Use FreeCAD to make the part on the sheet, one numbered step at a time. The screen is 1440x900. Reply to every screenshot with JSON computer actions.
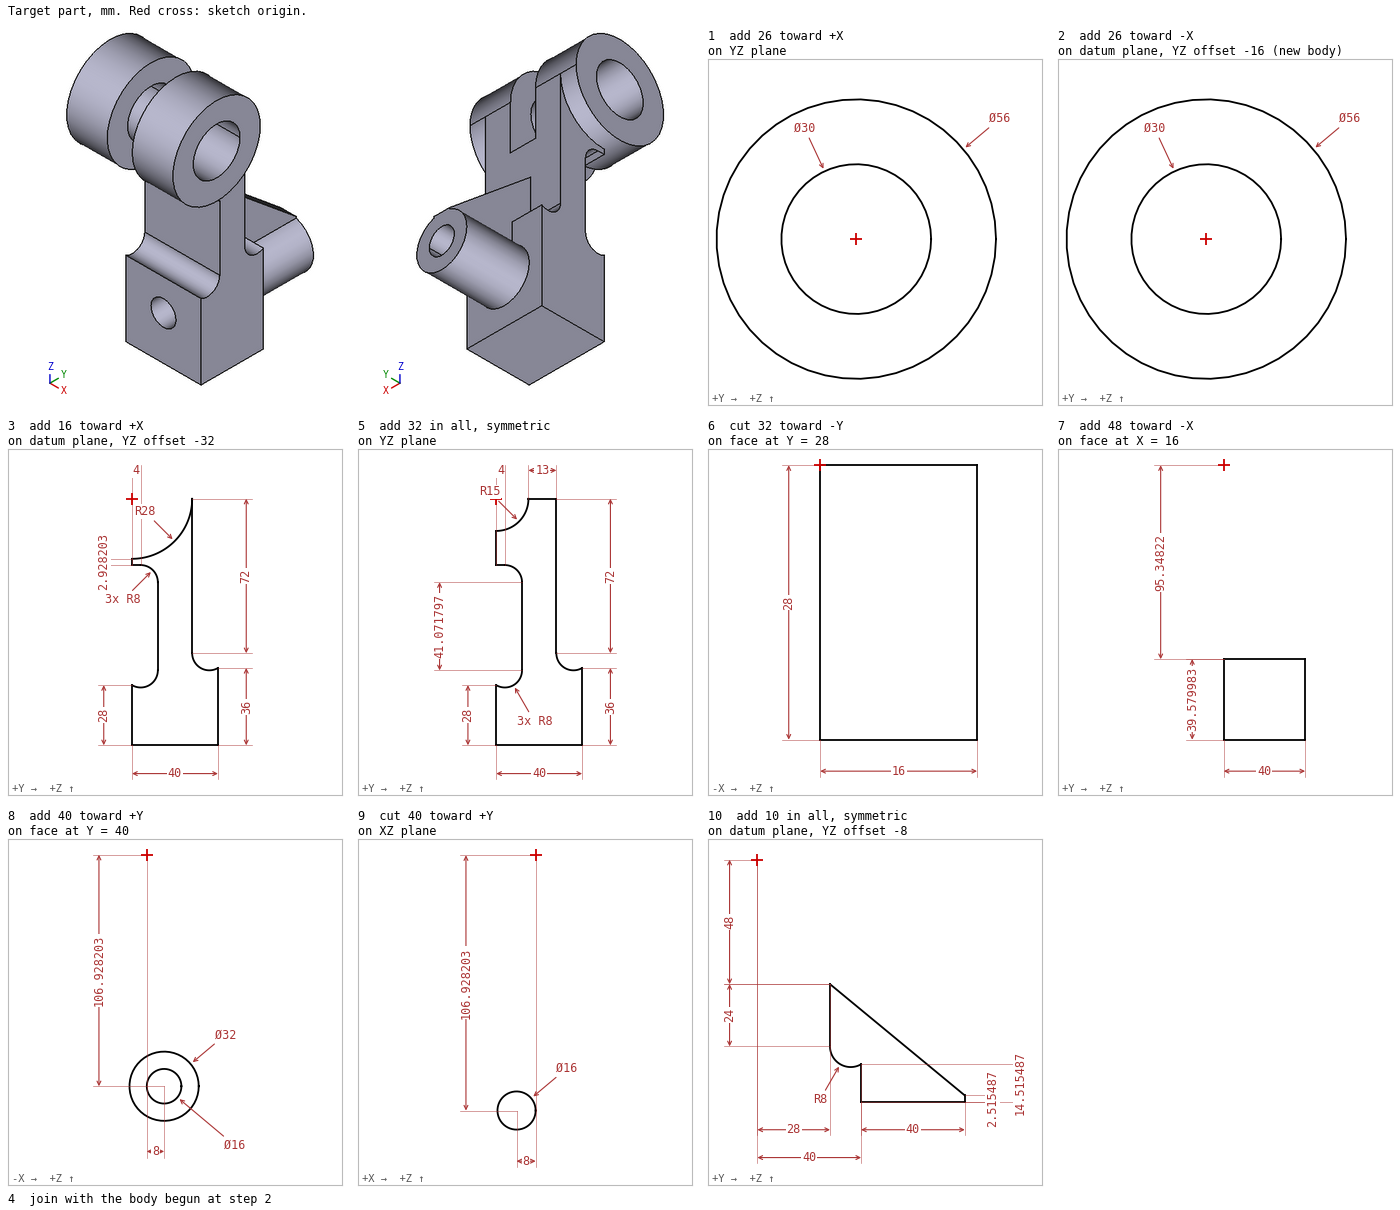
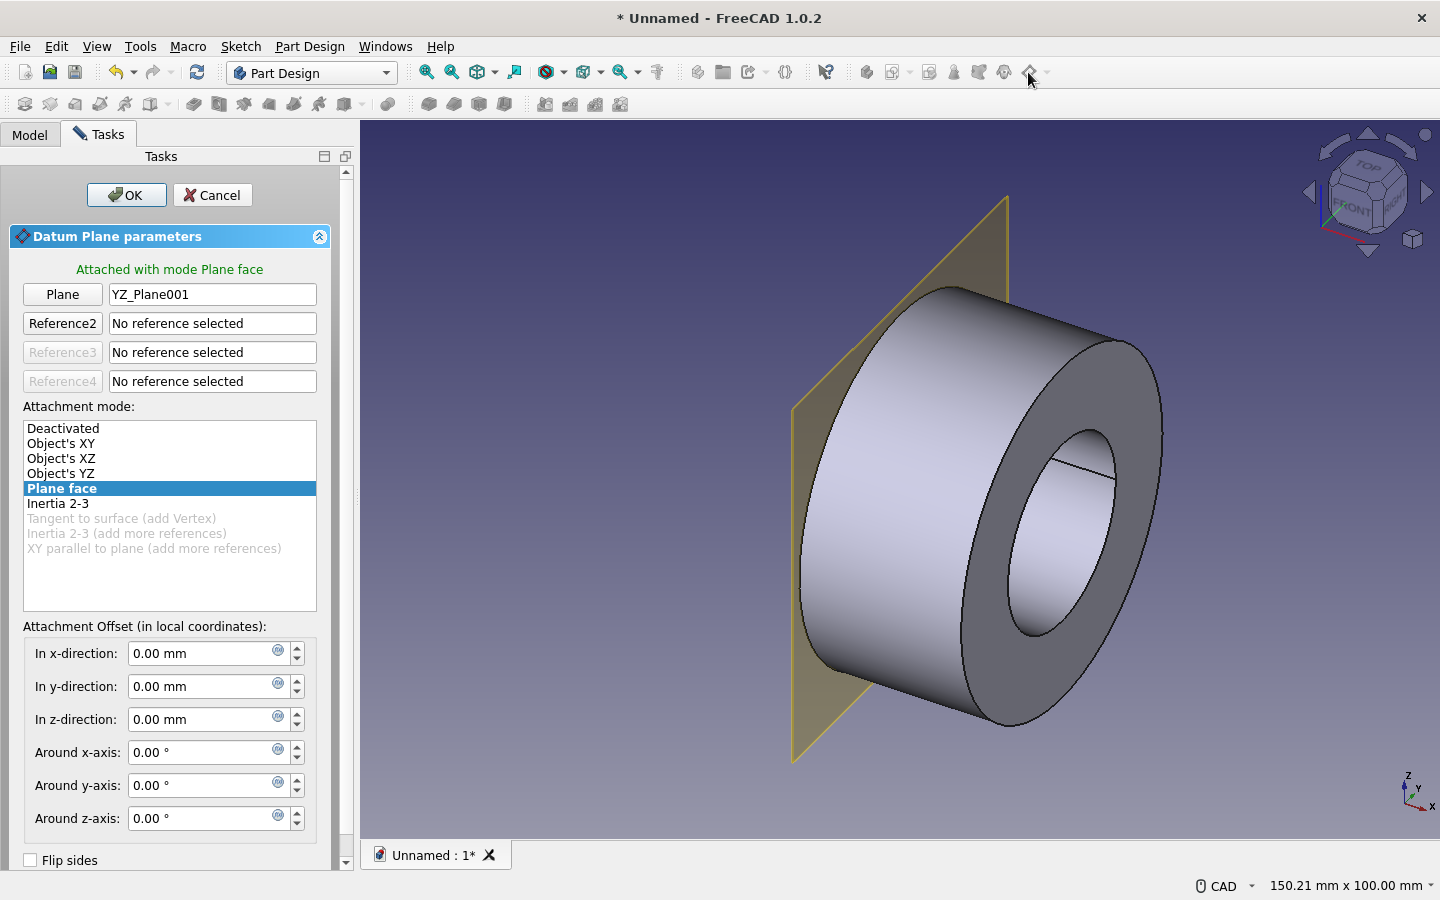
{"action": "triple_click", "coordinate": [210, 720]}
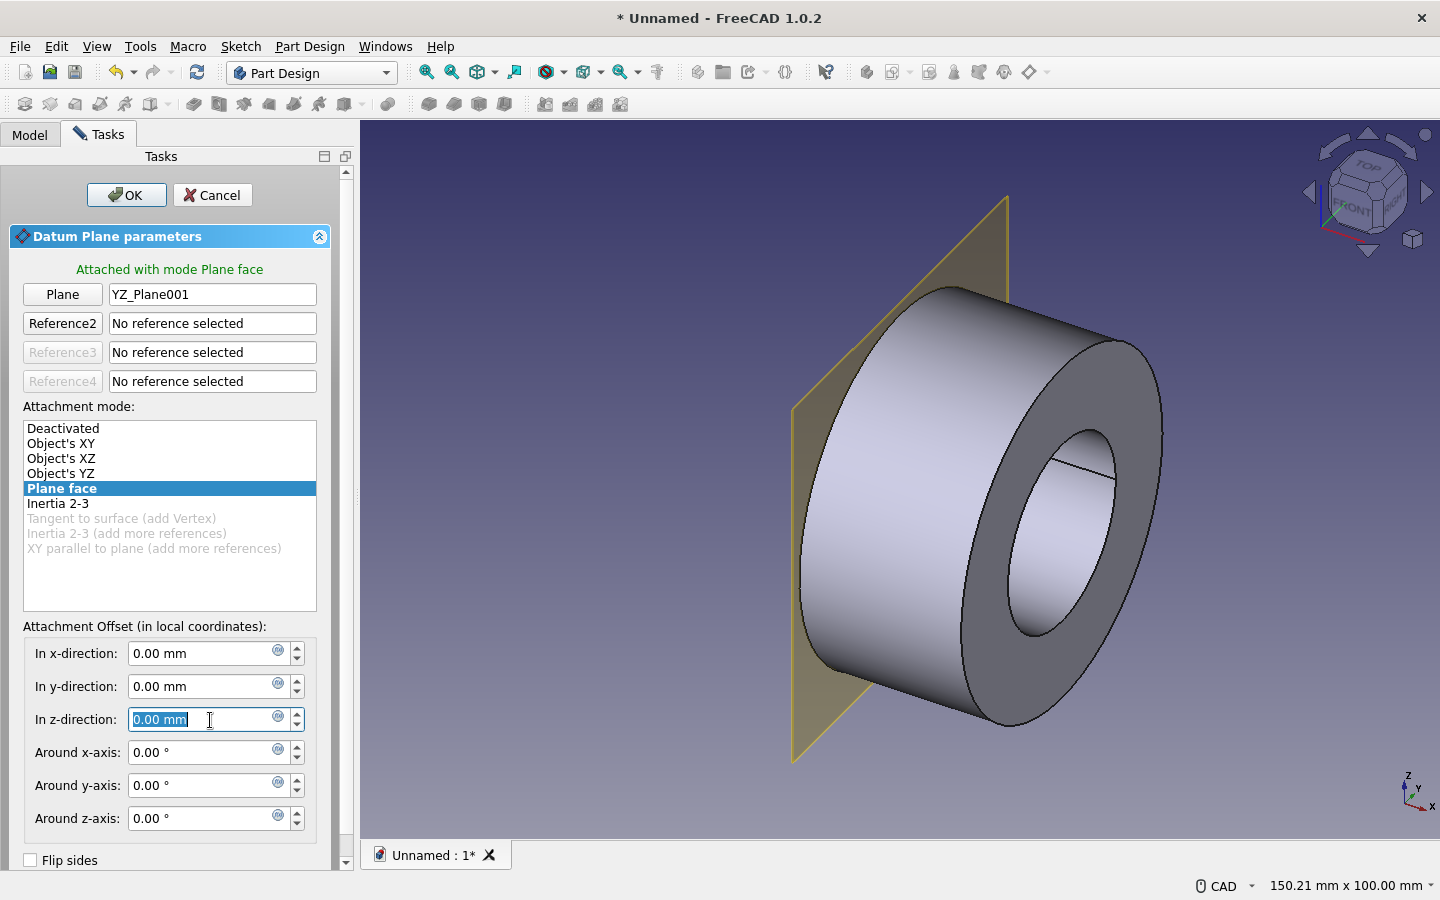
{"action": "type", "text": "-16"}
{"action": "key", "text": "Tab"}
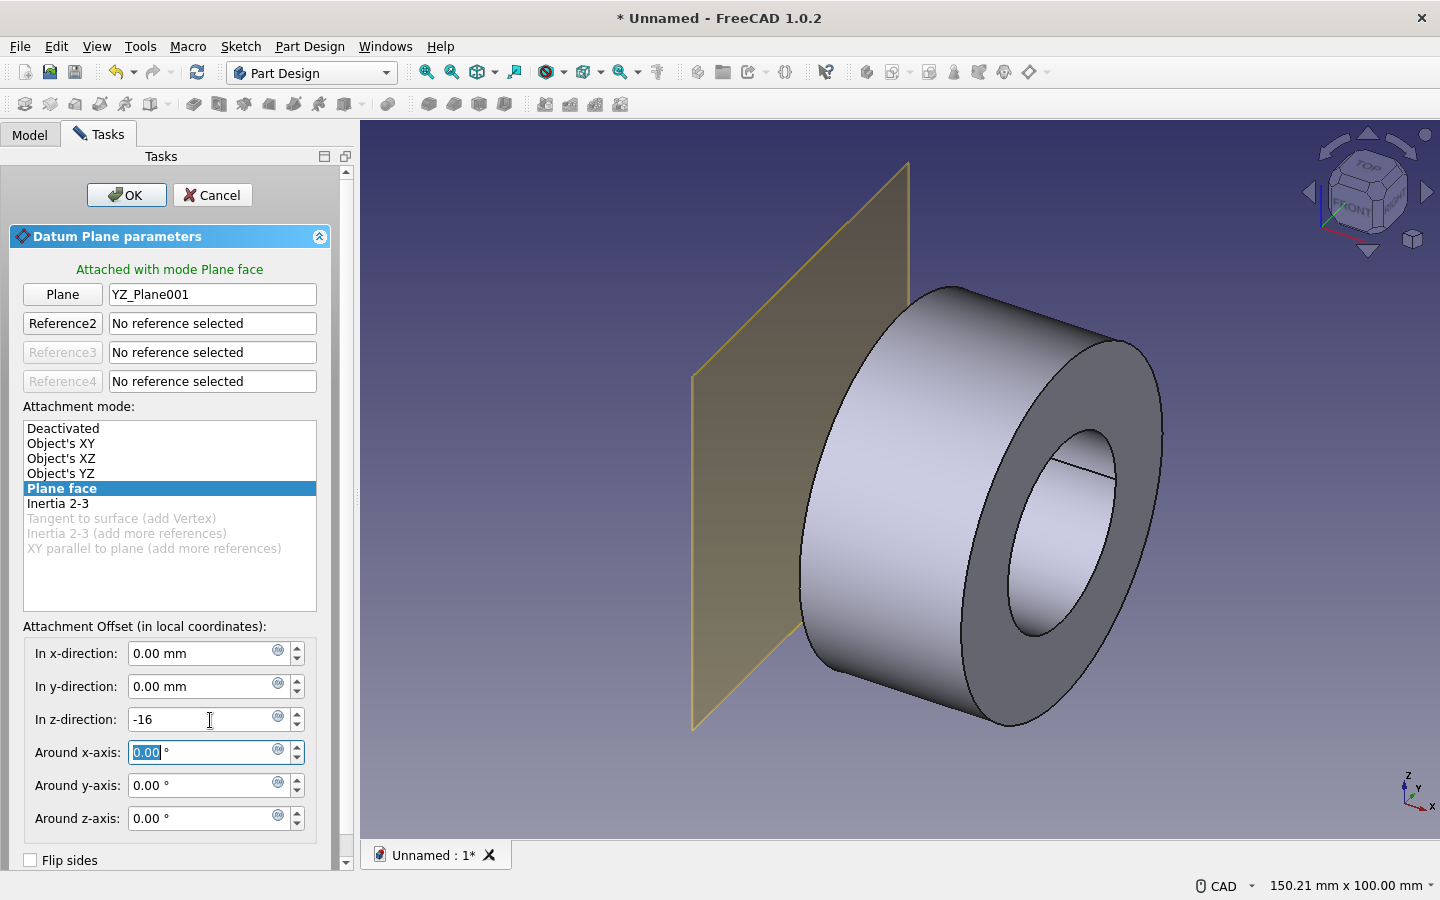
{"action": "left_click", "coordinate": [127, 195]}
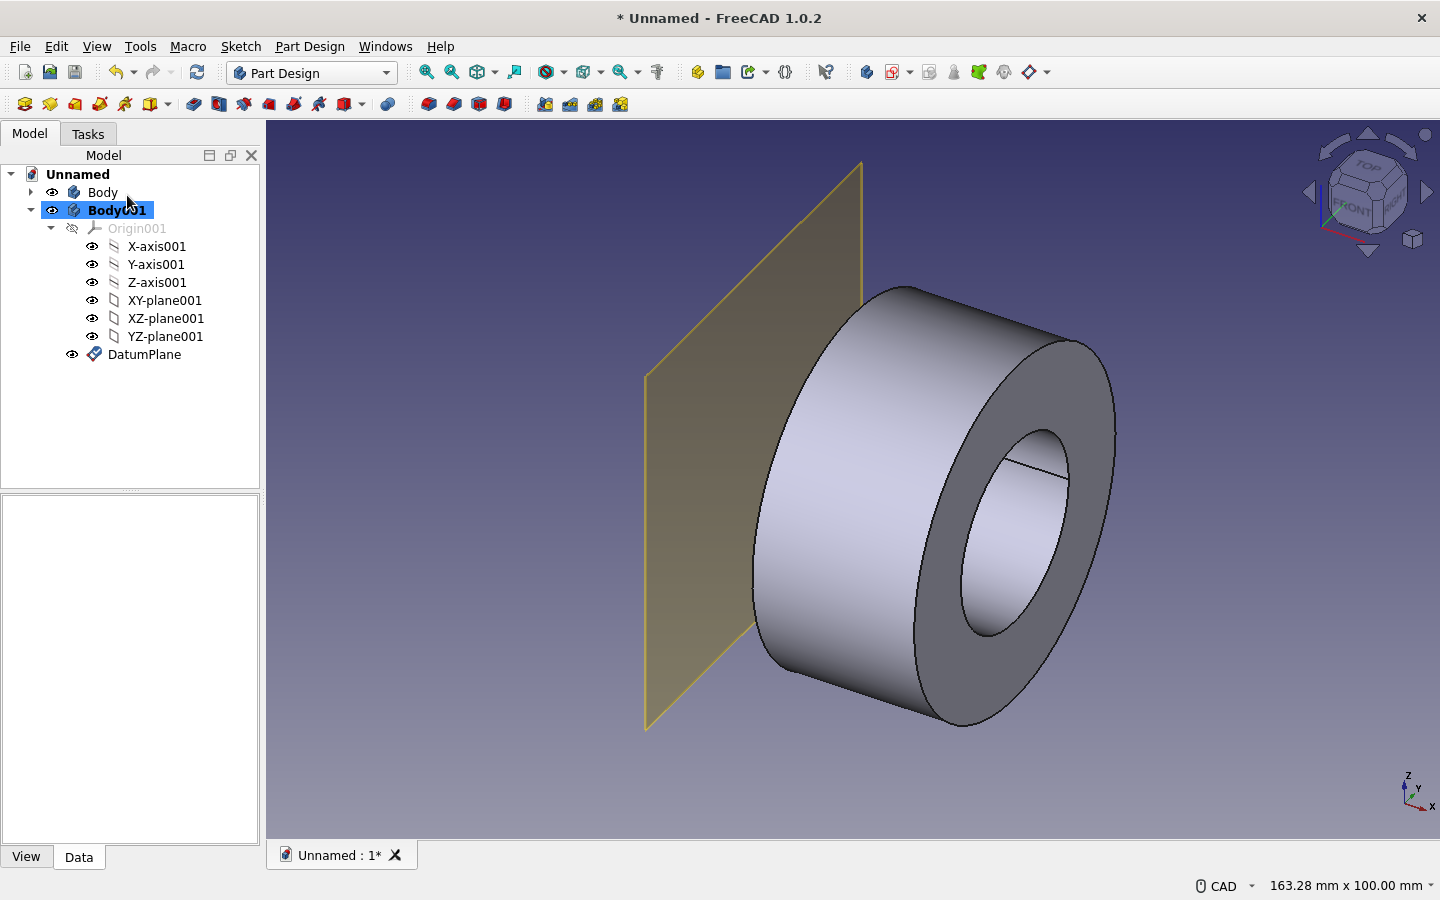
{"action": "left_click", "coordinate": [117, 354]}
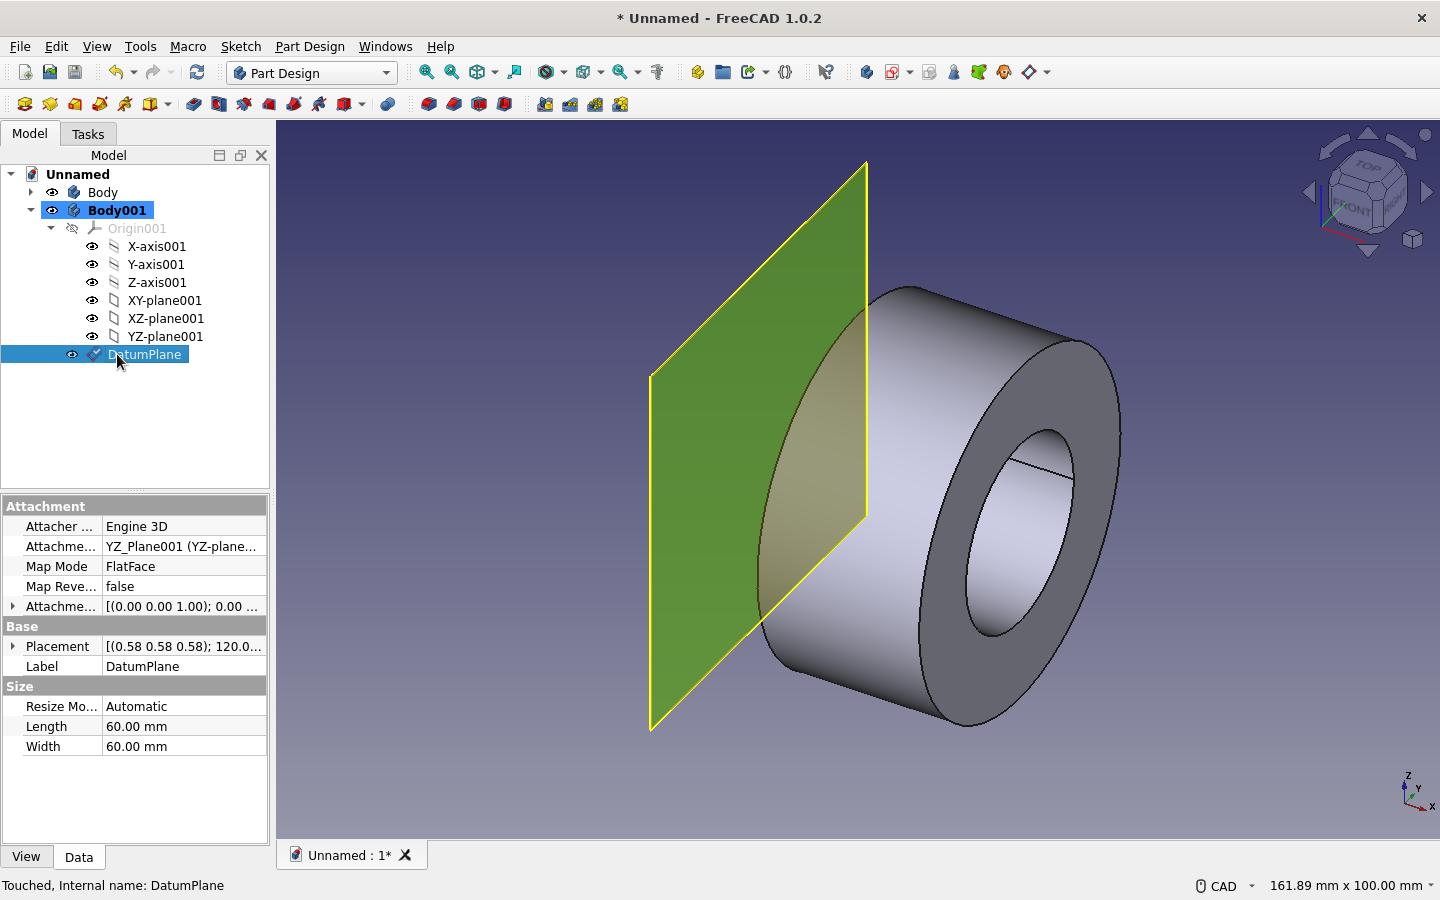
{"action": "left_click", "coordinate": [892, 72]}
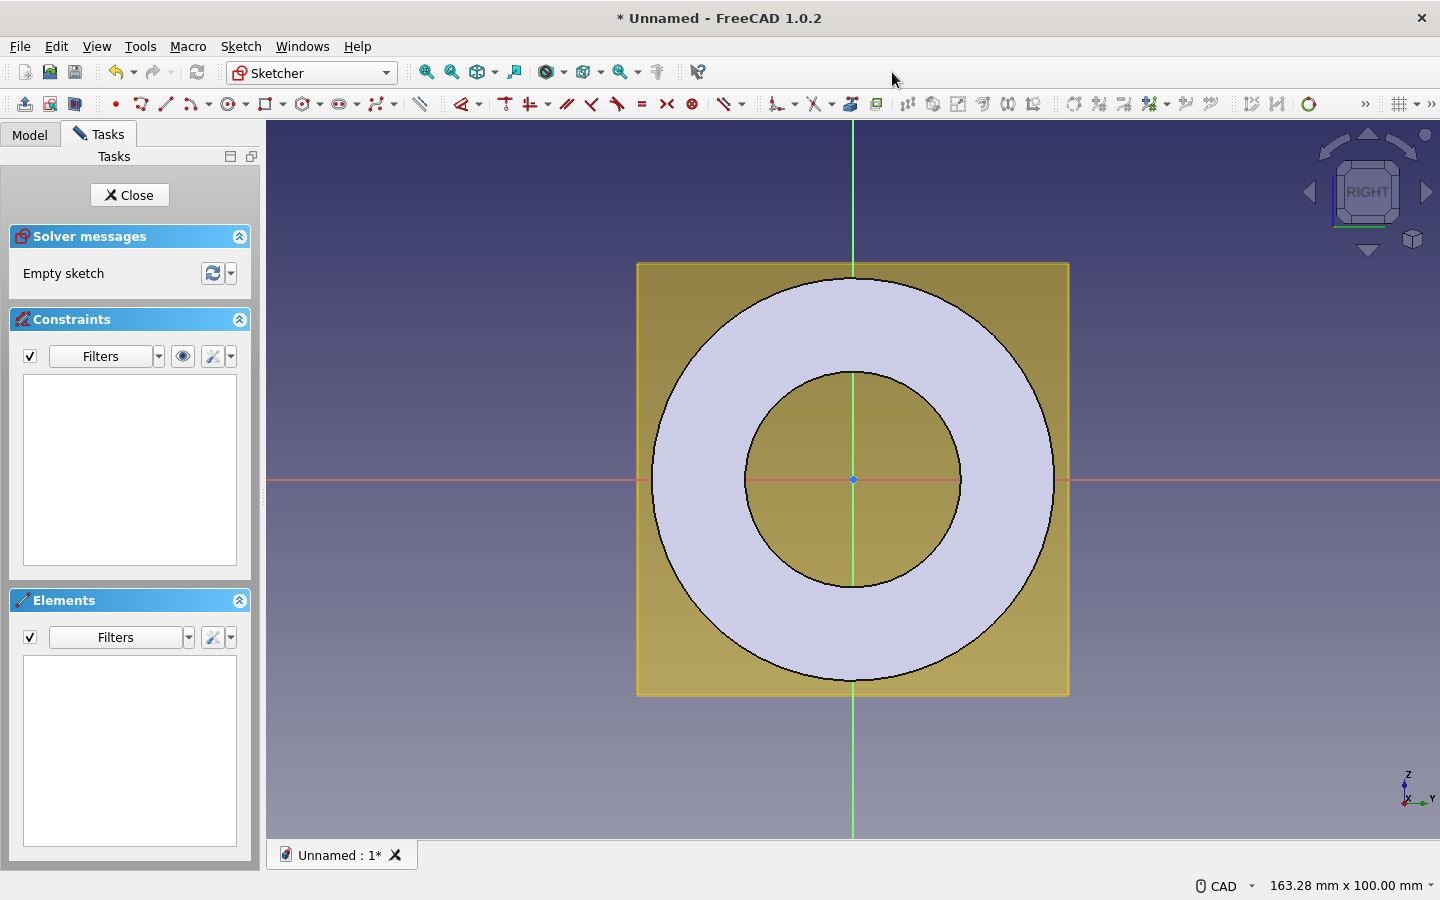
{"action": "key", "text": "g c"}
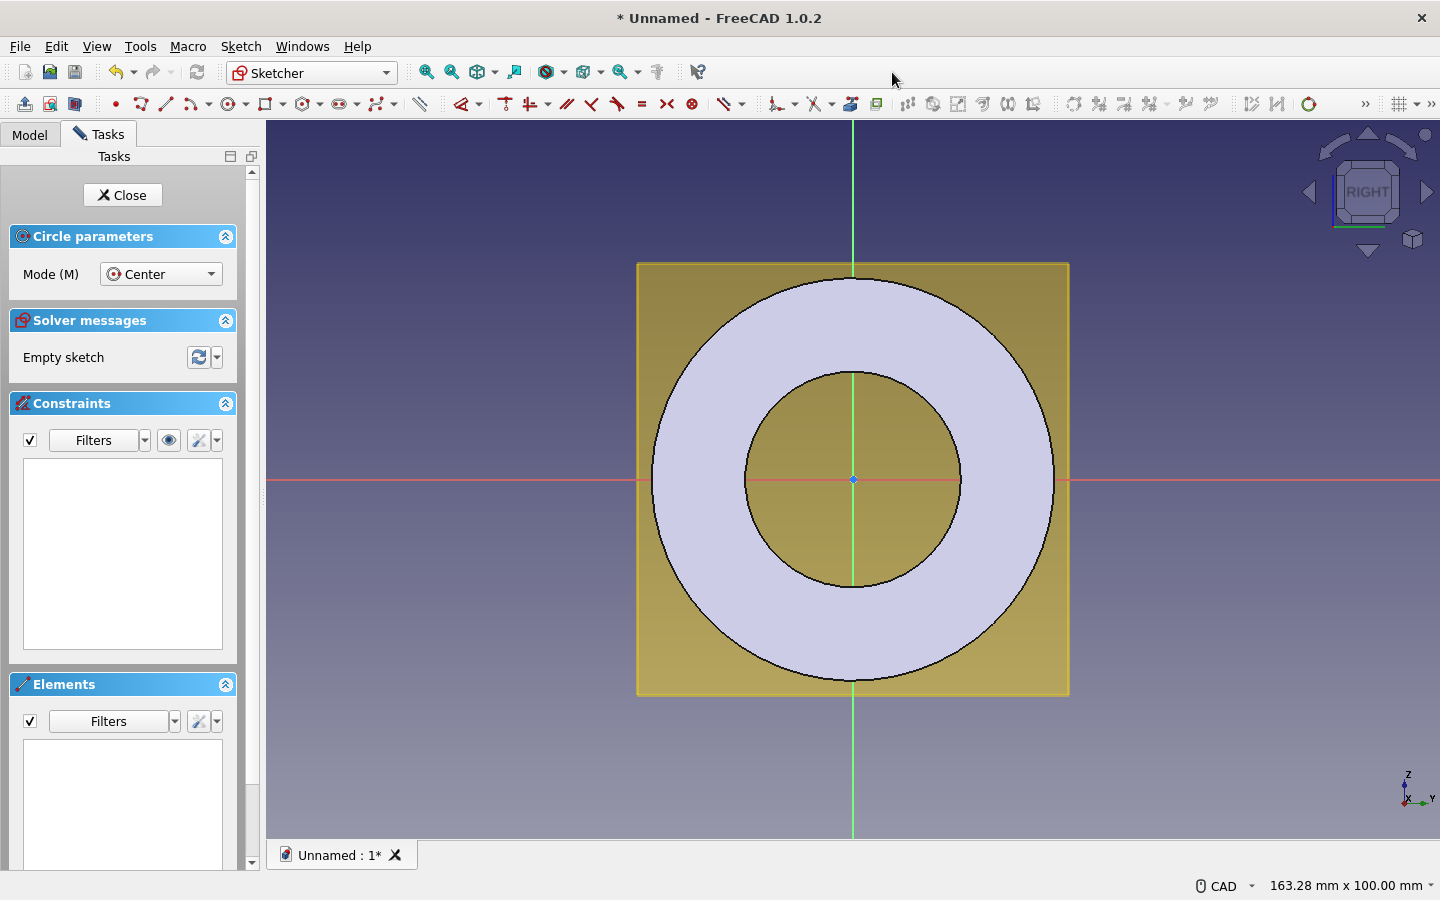
{"action": "left_click", "coordinate": [853, 480]}
{"action": "left_click", "coordinate": [995, 337]}